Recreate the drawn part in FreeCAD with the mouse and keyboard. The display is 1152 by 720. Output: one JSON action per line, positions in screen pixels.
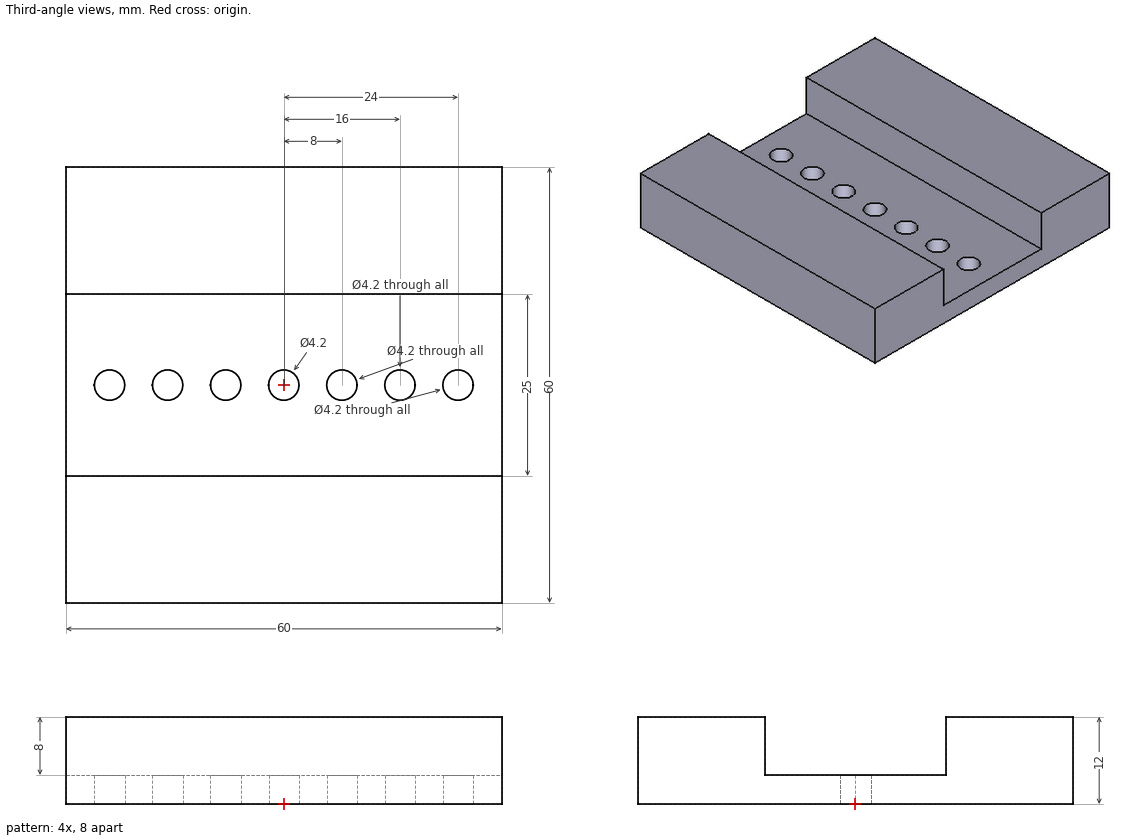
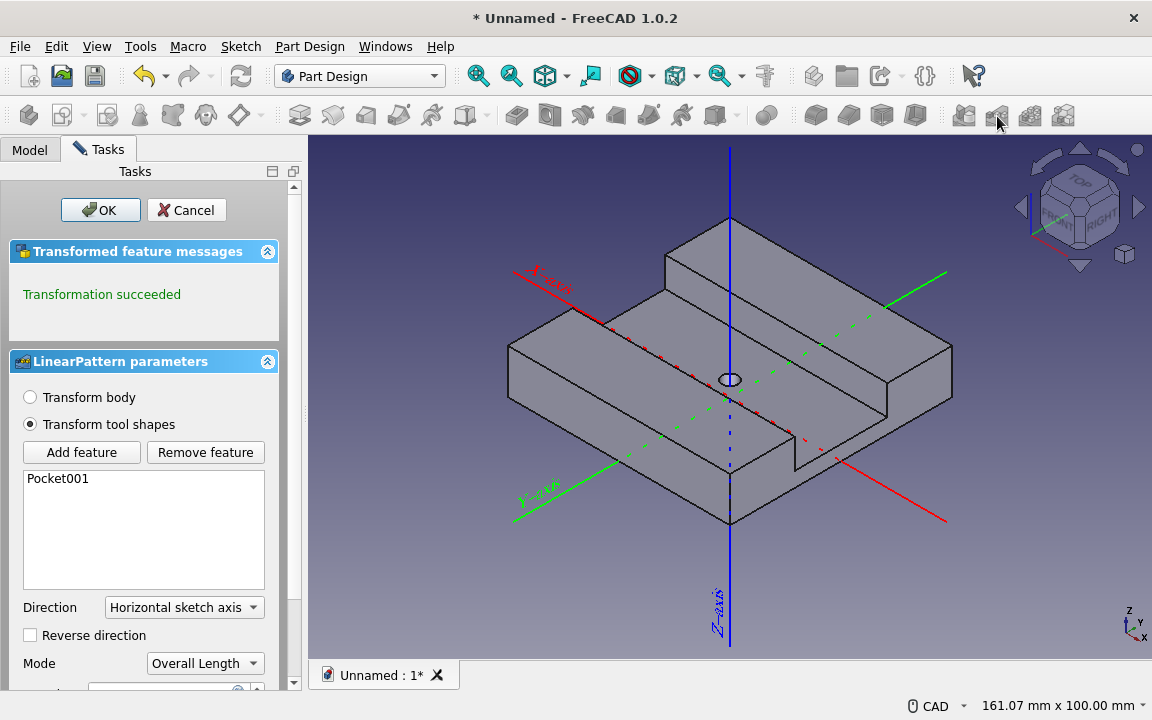
{"action": "left_click", "coordinate": [185, 608]}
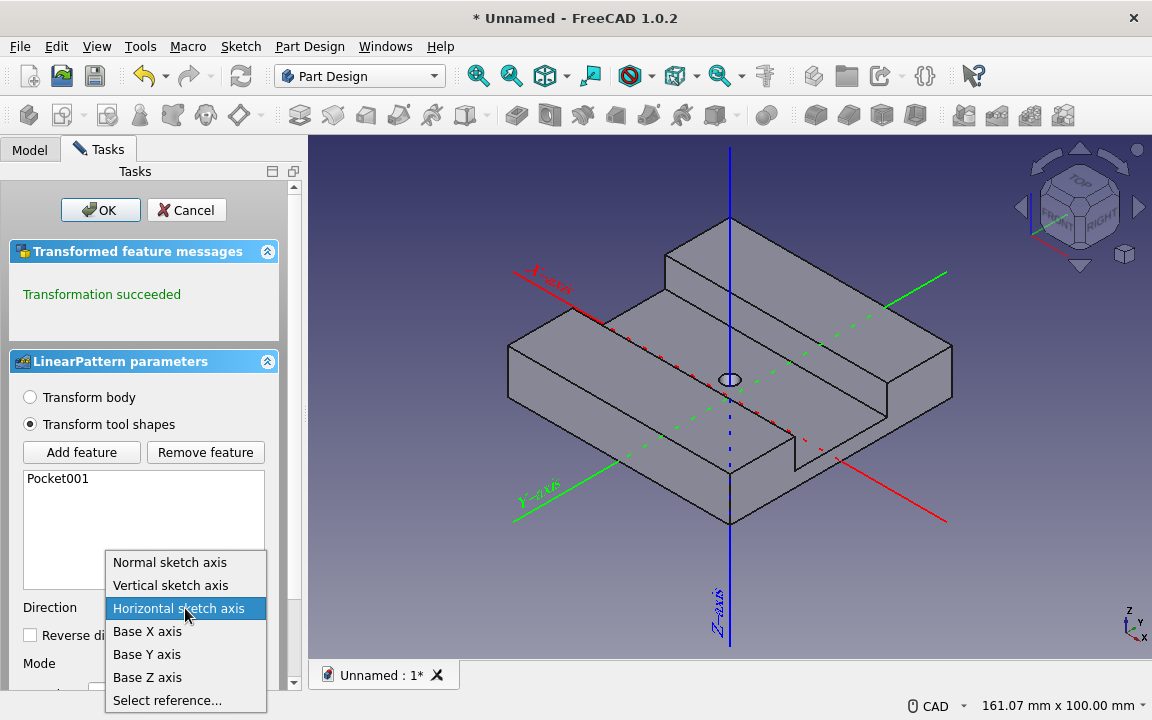
{"action": "left_click", "coordinate": [184, 632]}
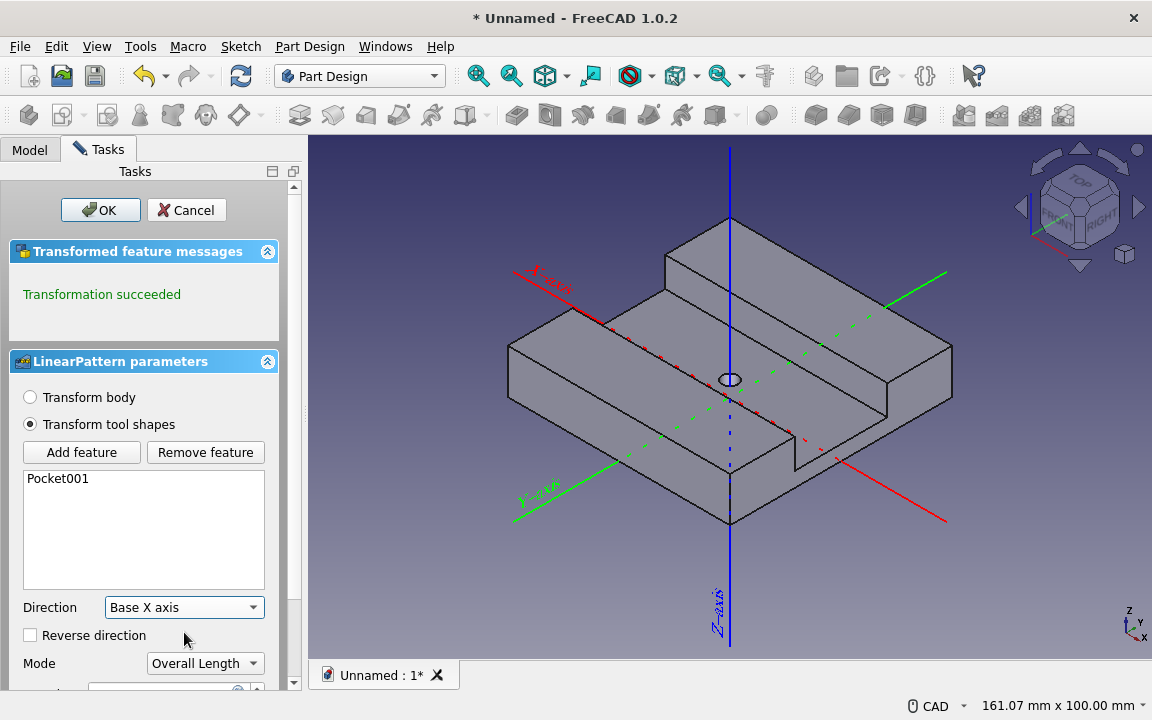
{"action": "left_click", "coordinate": [206, 664]}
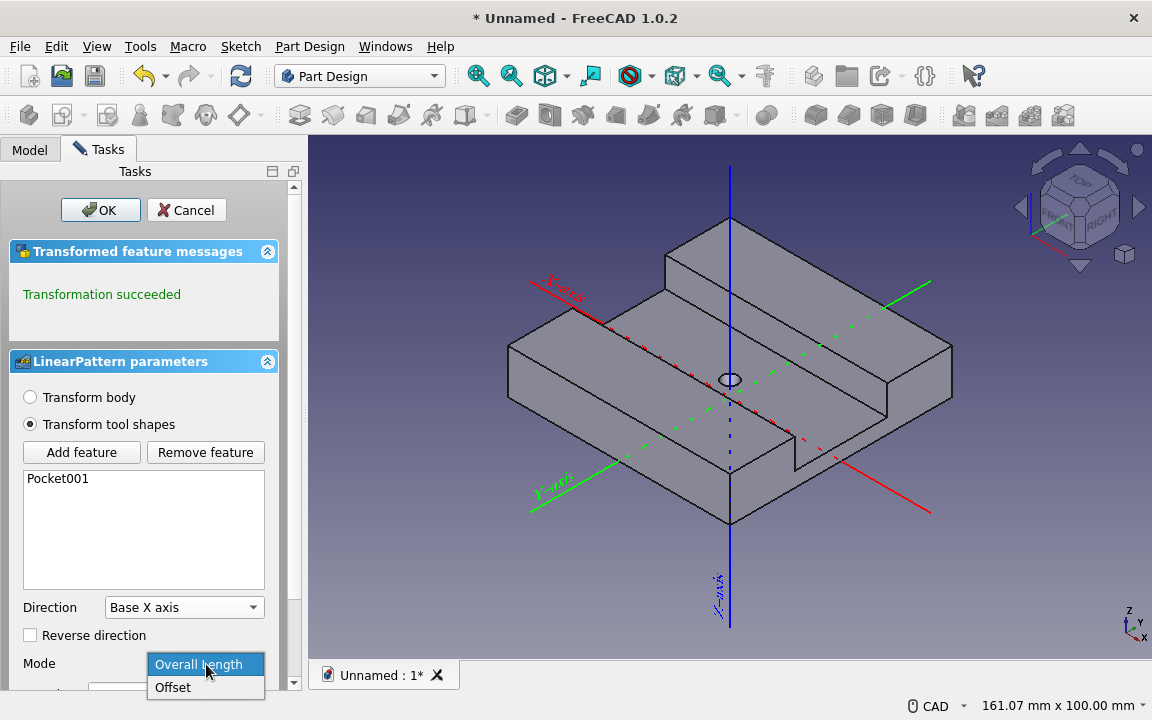
{"action": "left_click", "coordinate": [204, 688]}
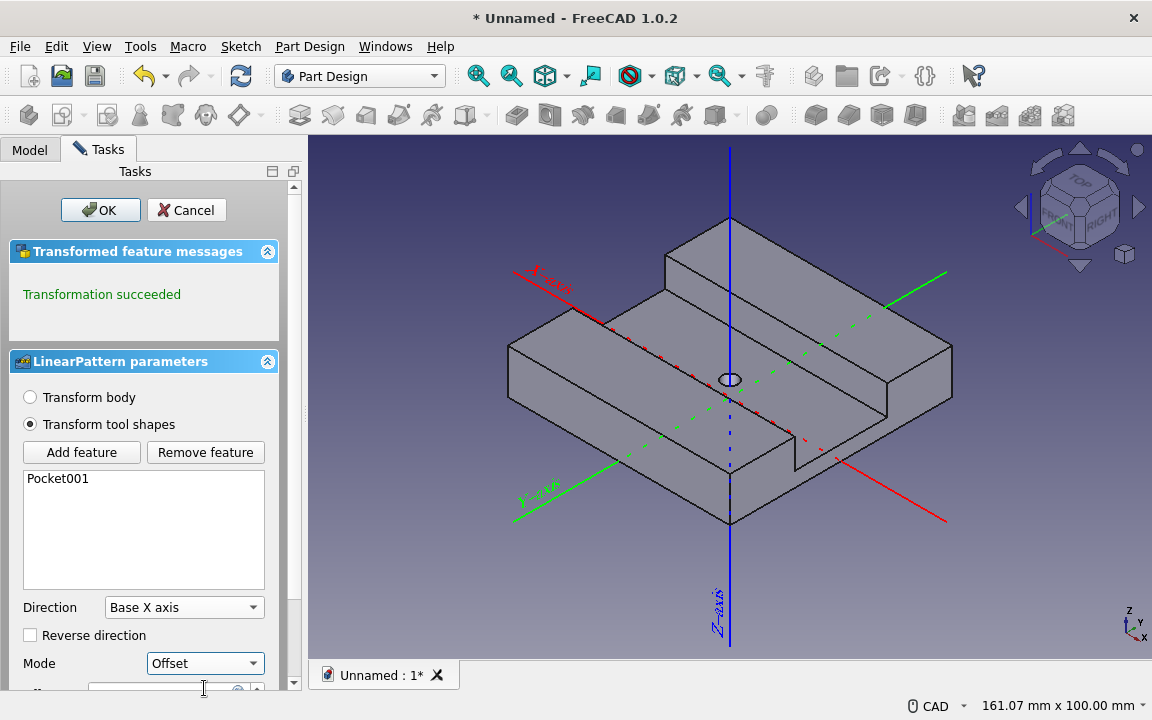
{"action": "scroll", "coordinate": [294, 436], "scroll_direction": "down", "scroll_amount": 2}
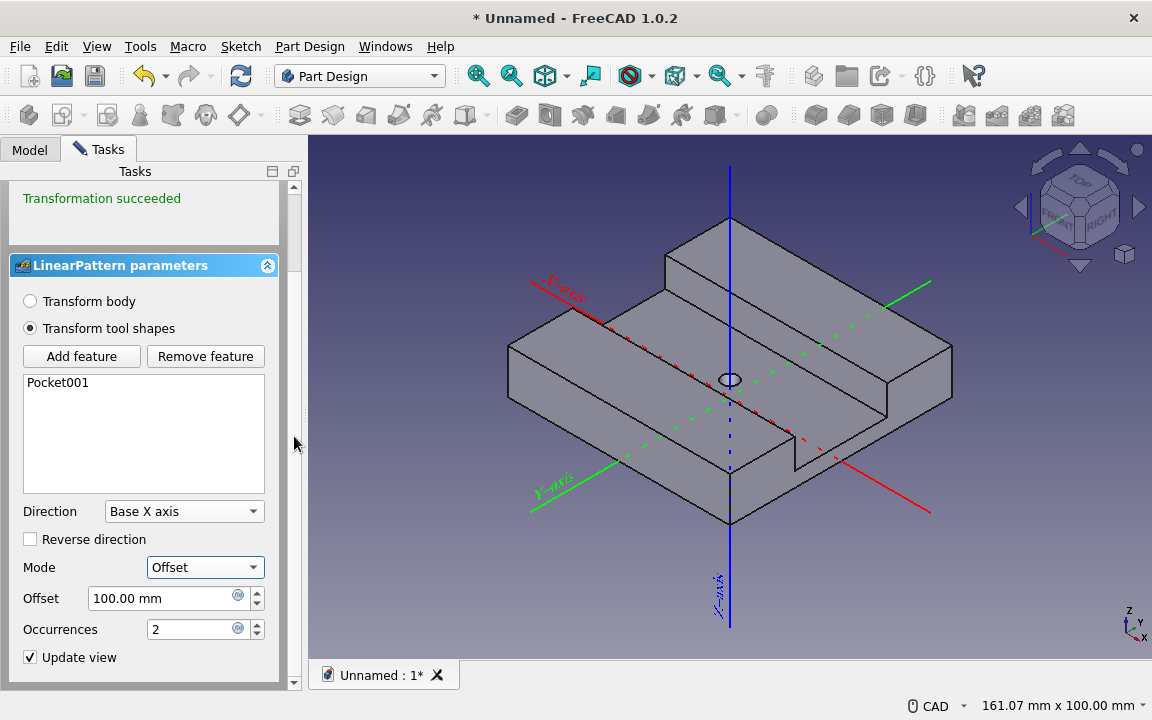
{"action": "triple_click", "coordinate": [170, 598]}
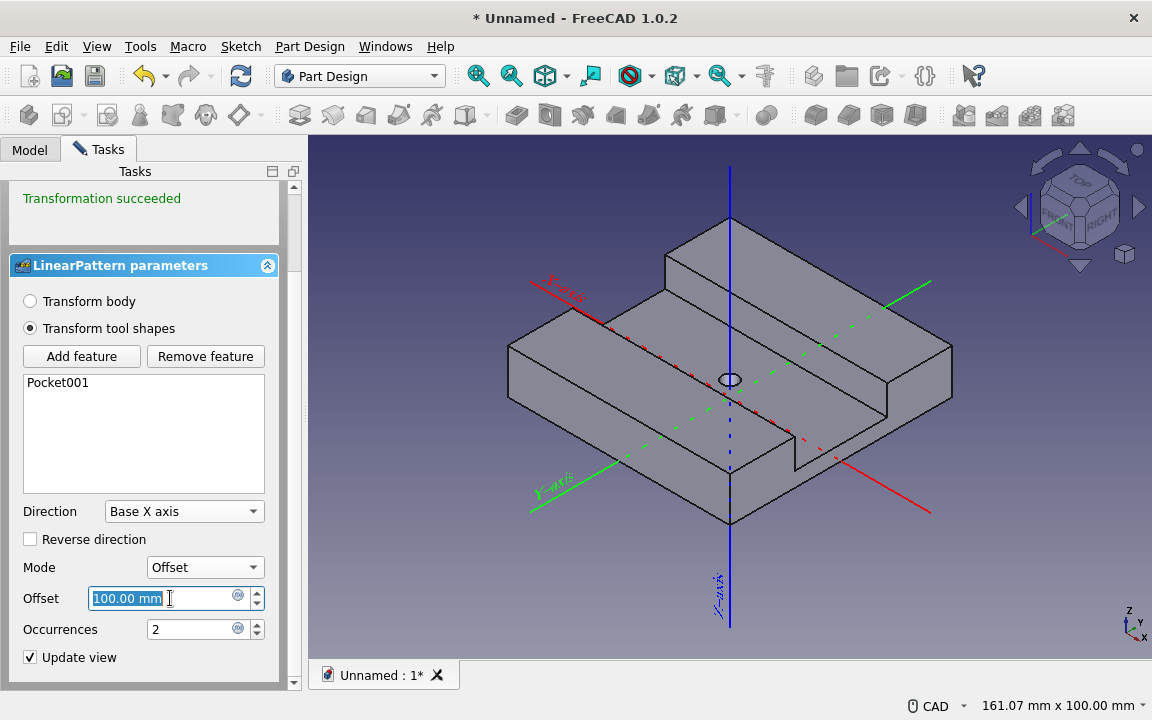
{"action": "type", "text": "8"}
{"action": "key", "text": "Tab"}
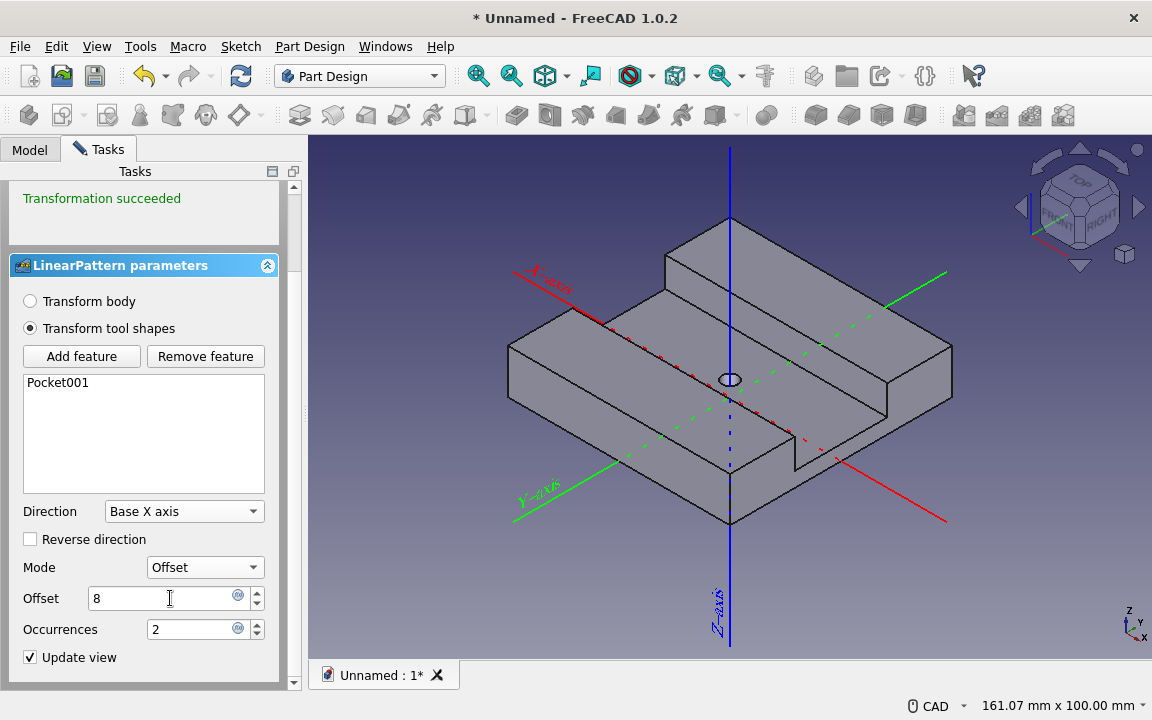
{"action": "triple_click", "coordinate": [199, 630]}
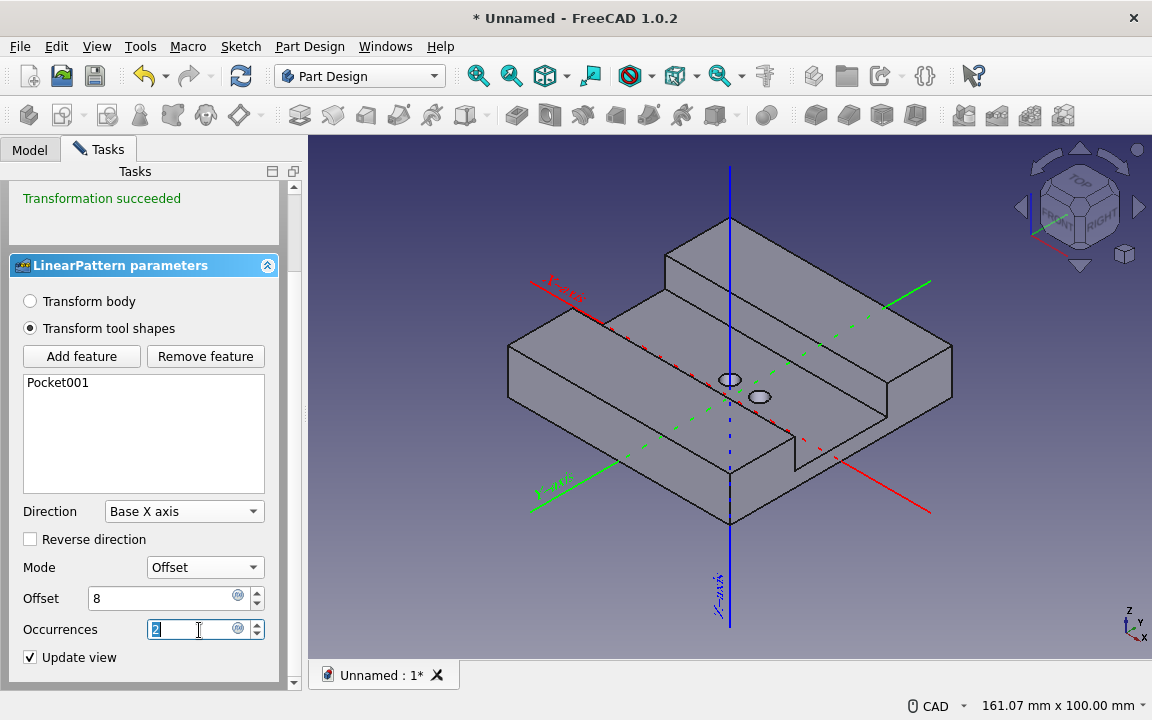
{"action": "type", "text": "4"}
{"action": "key", "text": "Tab"}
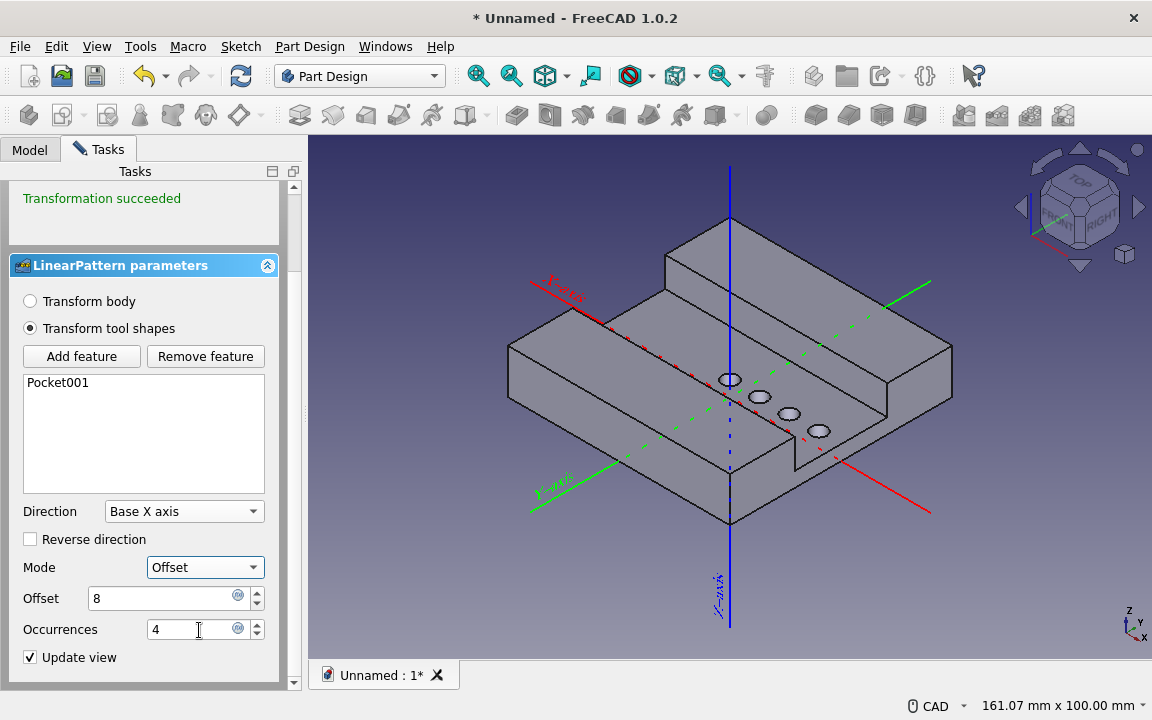
{"action": "left_click", "coordinate": [31, 539]}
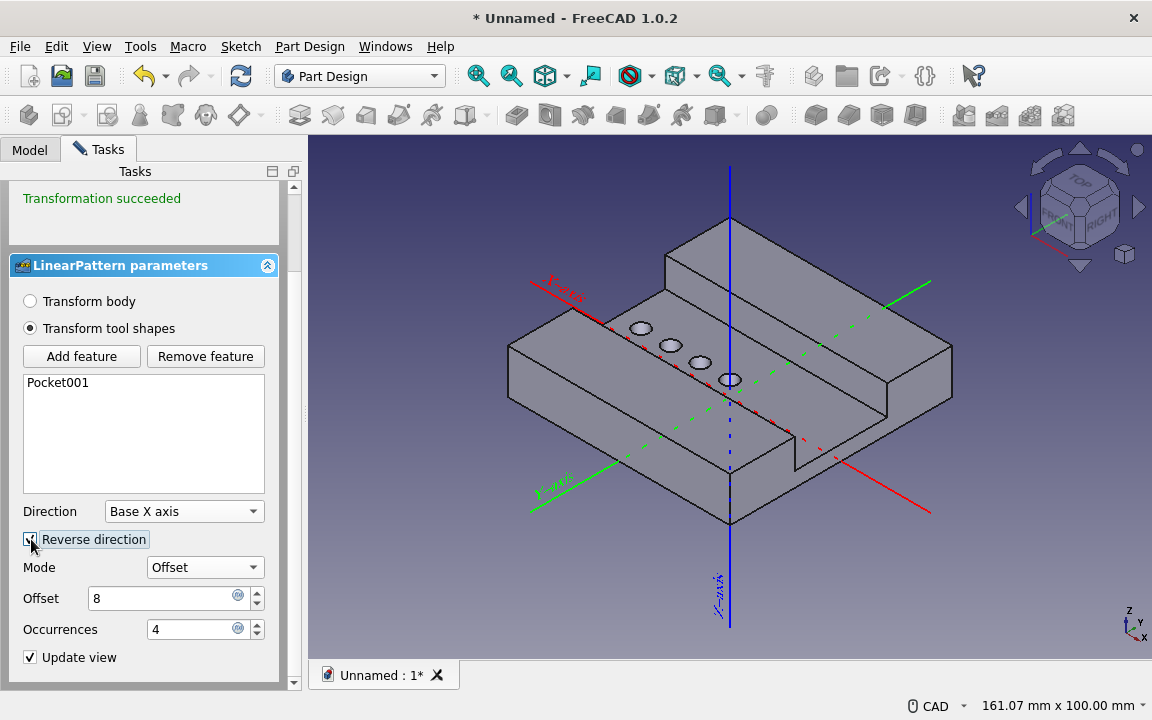
{"action": "scroll", "coordinate": [294, 436], "scroll_direction": "up", "scroll_amount": 3}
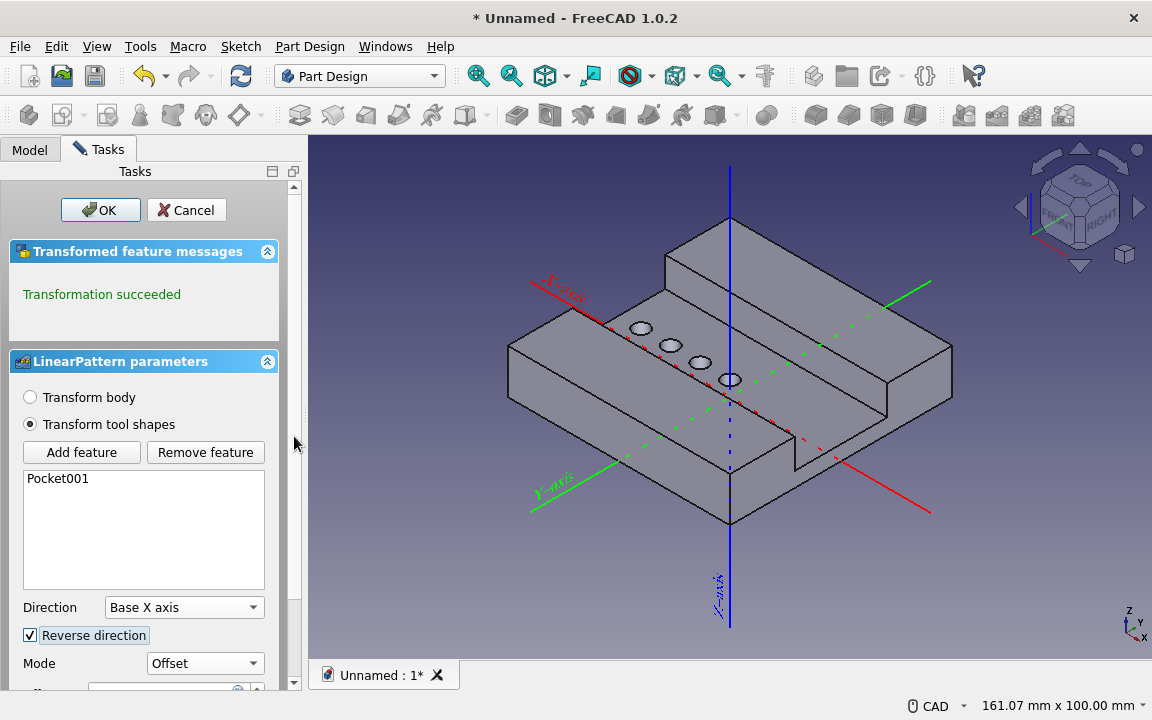
{"action": "left_click", "coordinate": [101, 210]}